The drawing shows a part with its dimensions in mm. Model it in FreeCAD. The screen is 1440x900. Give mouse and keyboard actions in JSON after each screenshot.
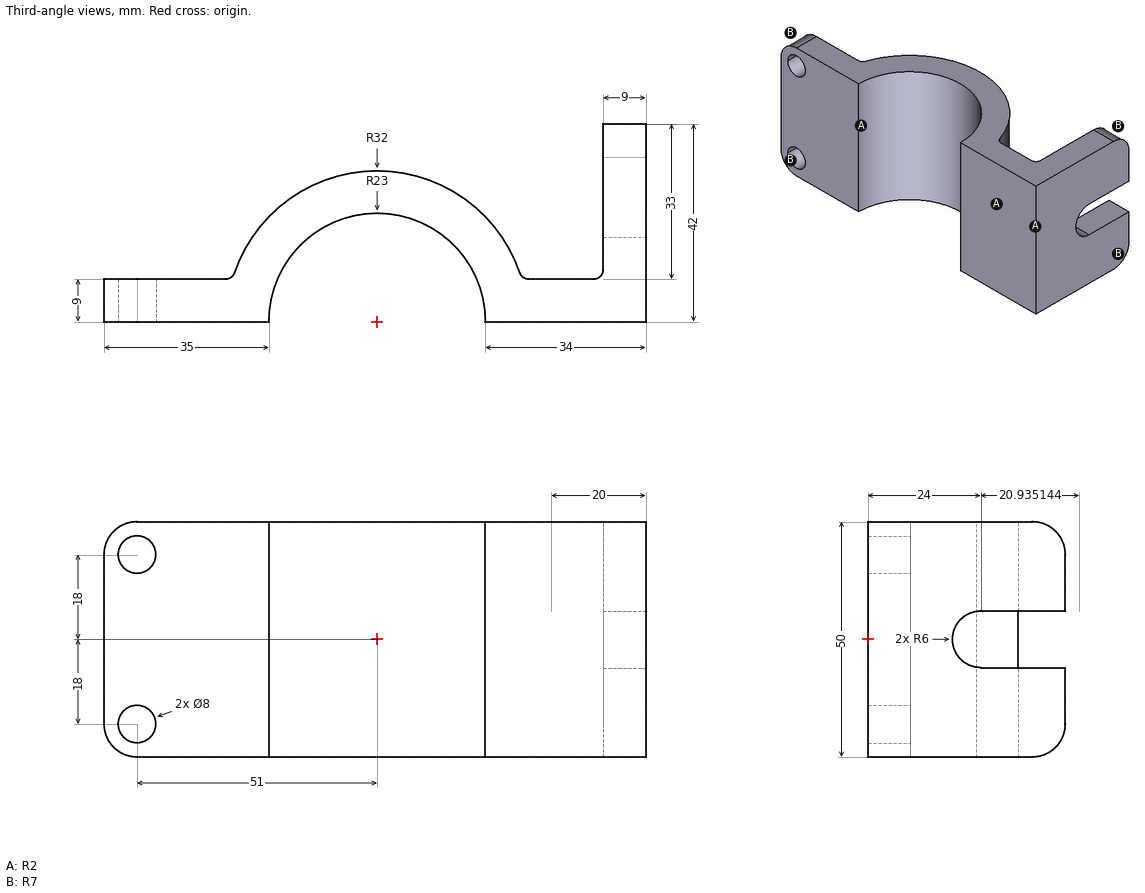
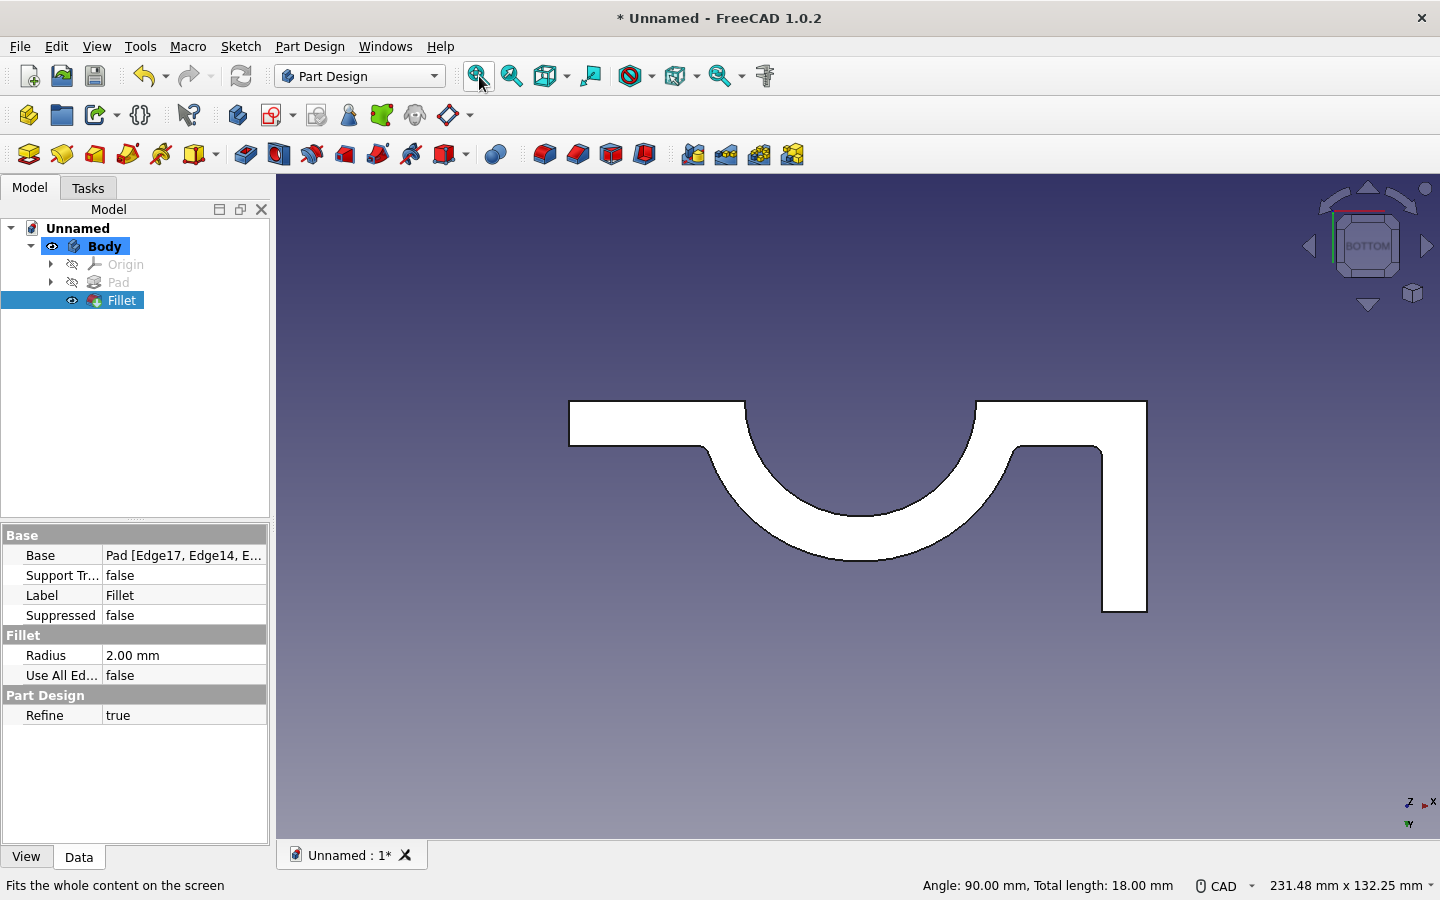
{"action": "left_click", "coordinate": [569, 423], "text": "ctrl"}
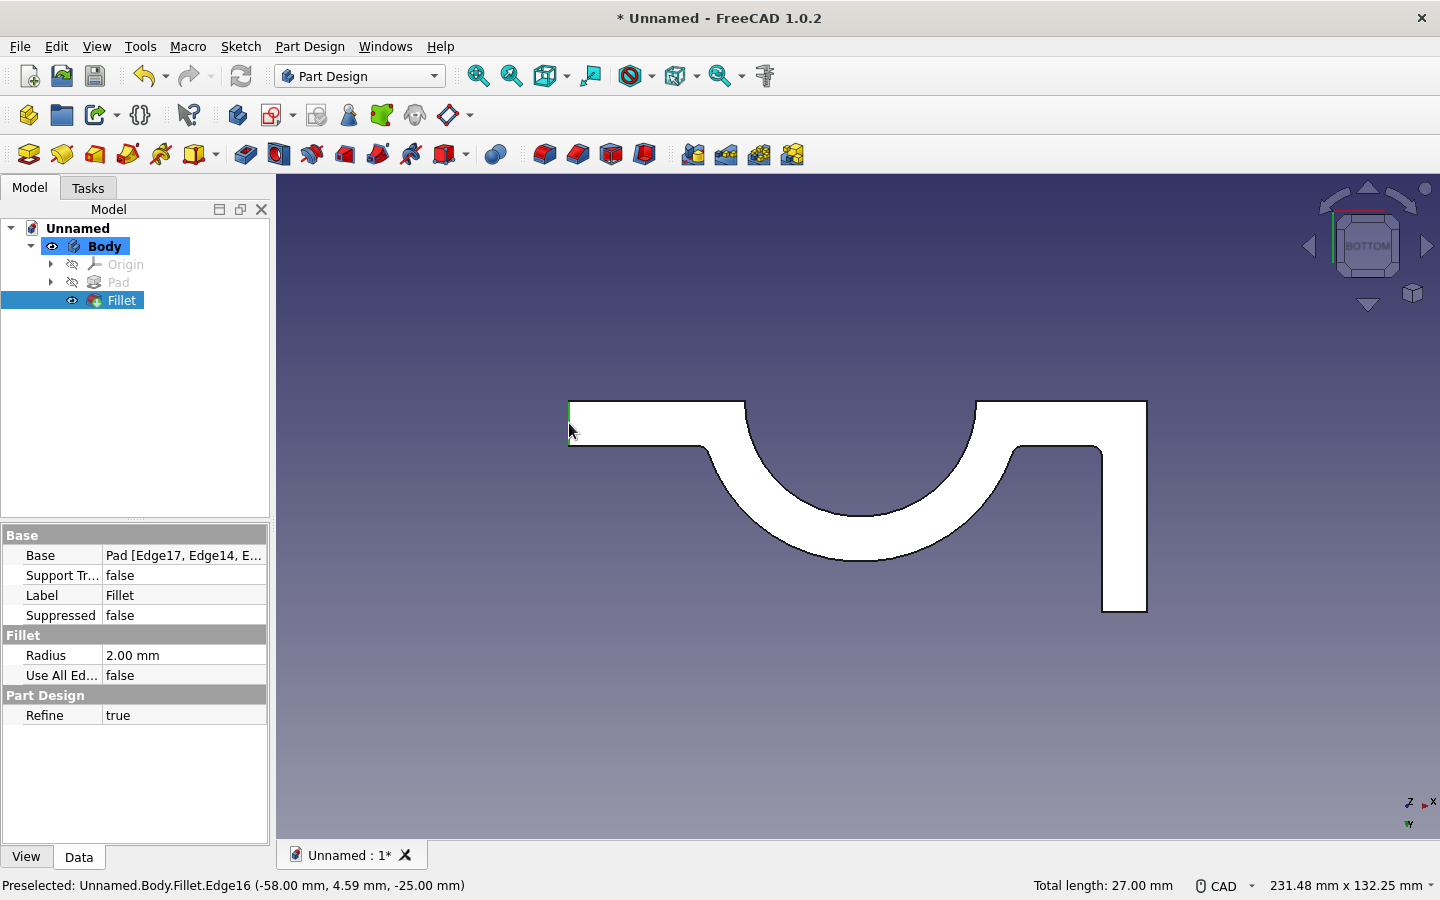
{"action": "left_click", "coordinate": [1125, 611], "text": "ctrl"}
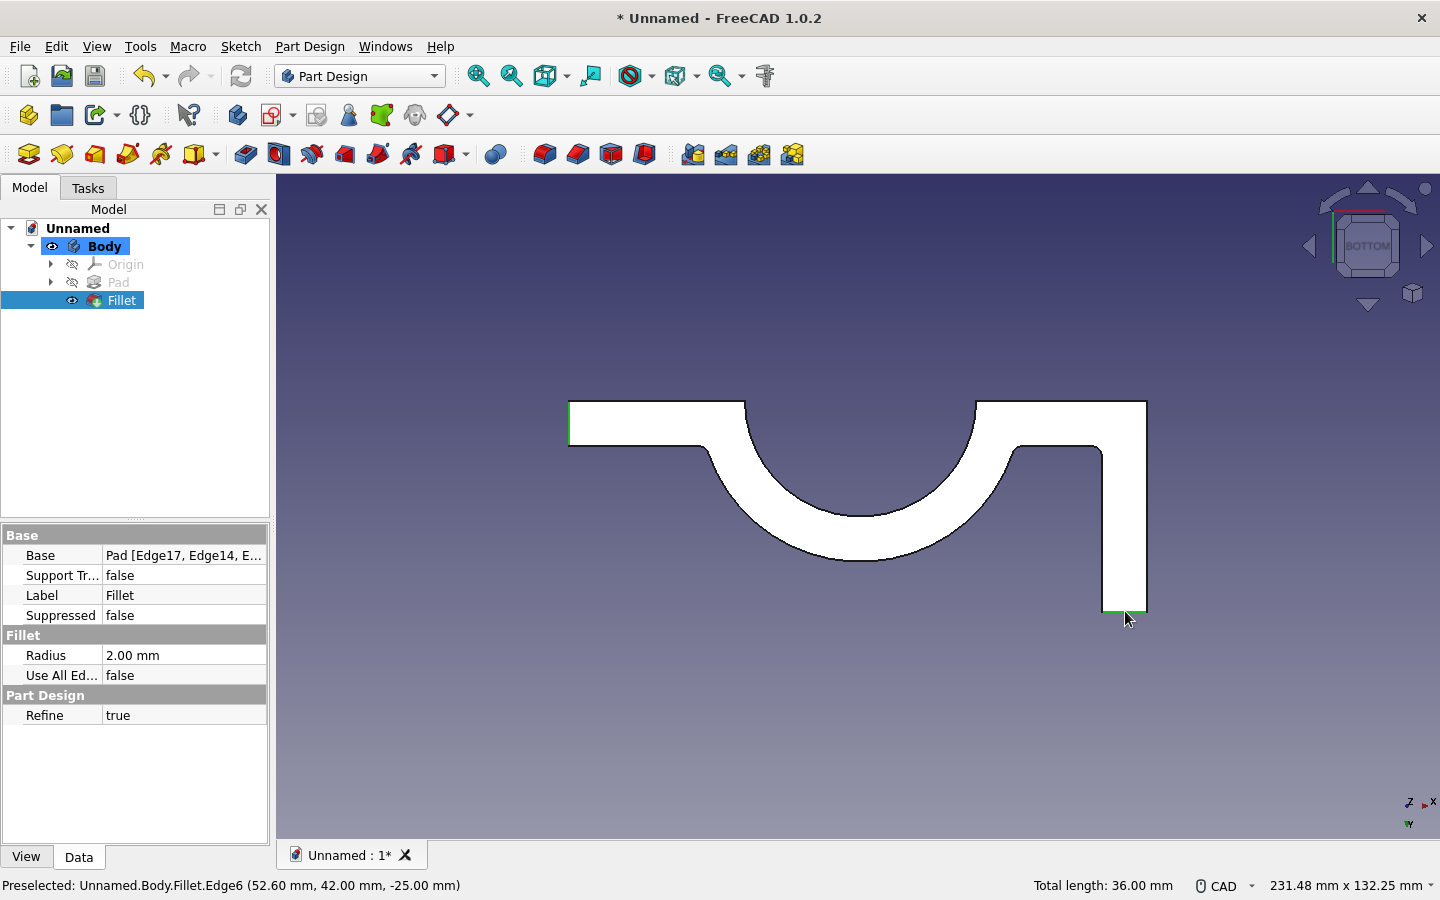
{"action": "left_click", "coordinate": [545, 154]}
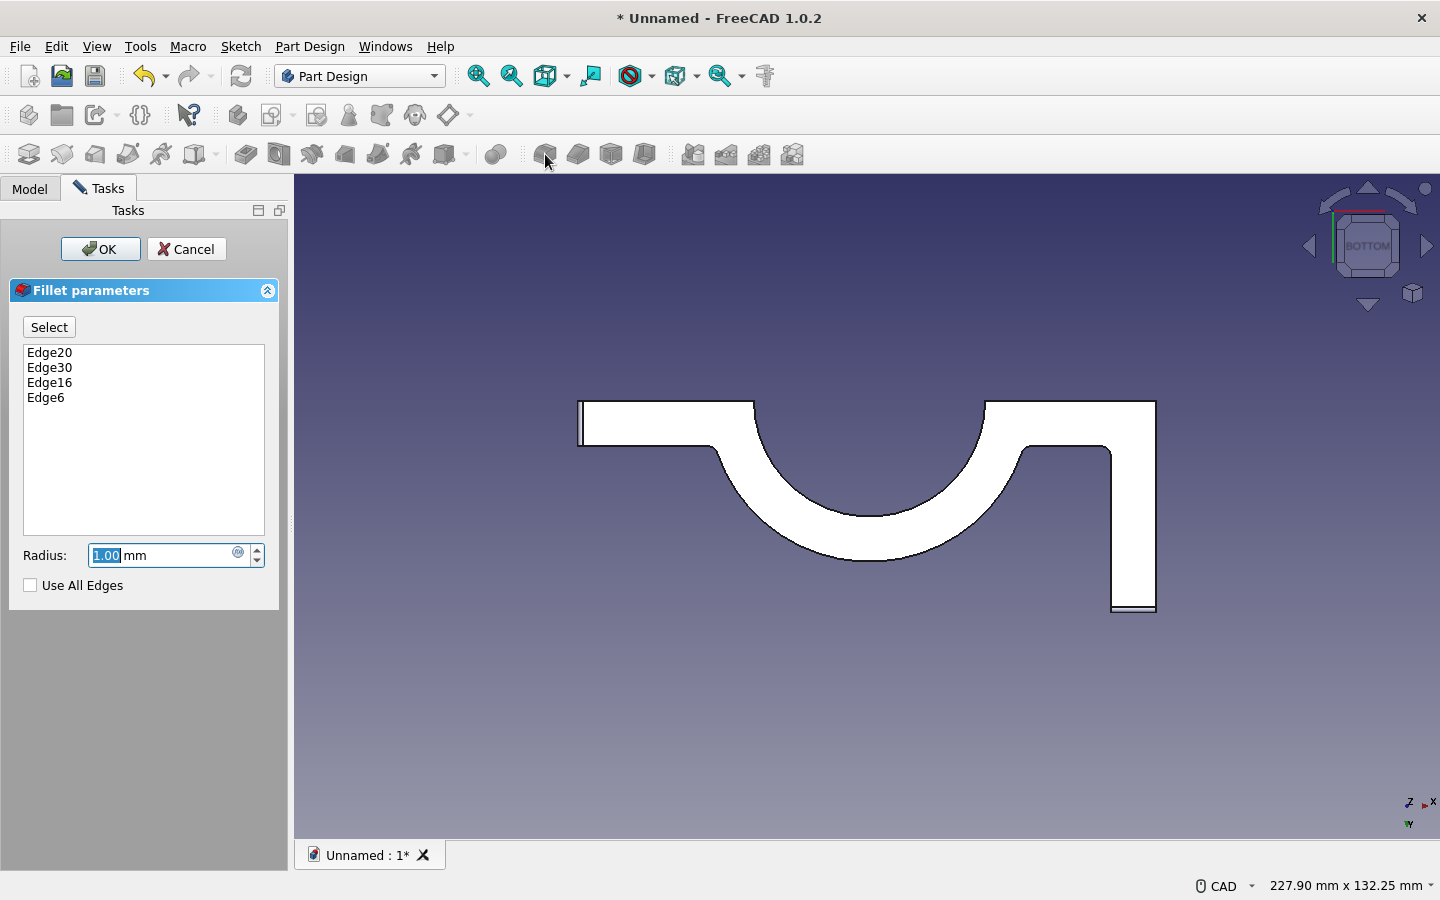
{"action": "type", "text": "7"}
{"action": "key", "text": "Tab"}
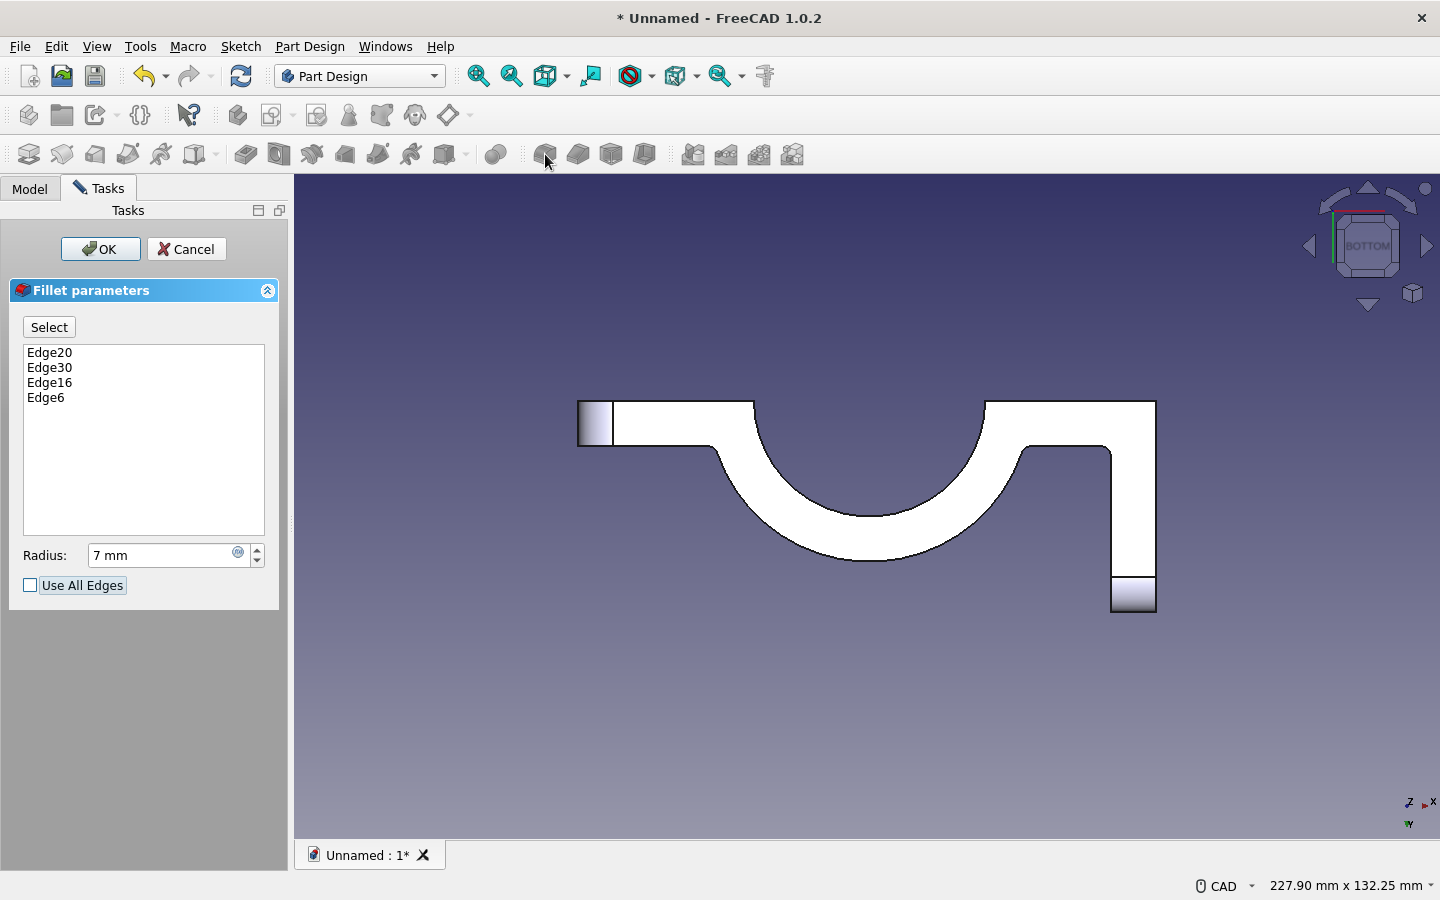
{"action": "left_click", "coordinate": [101, 249]}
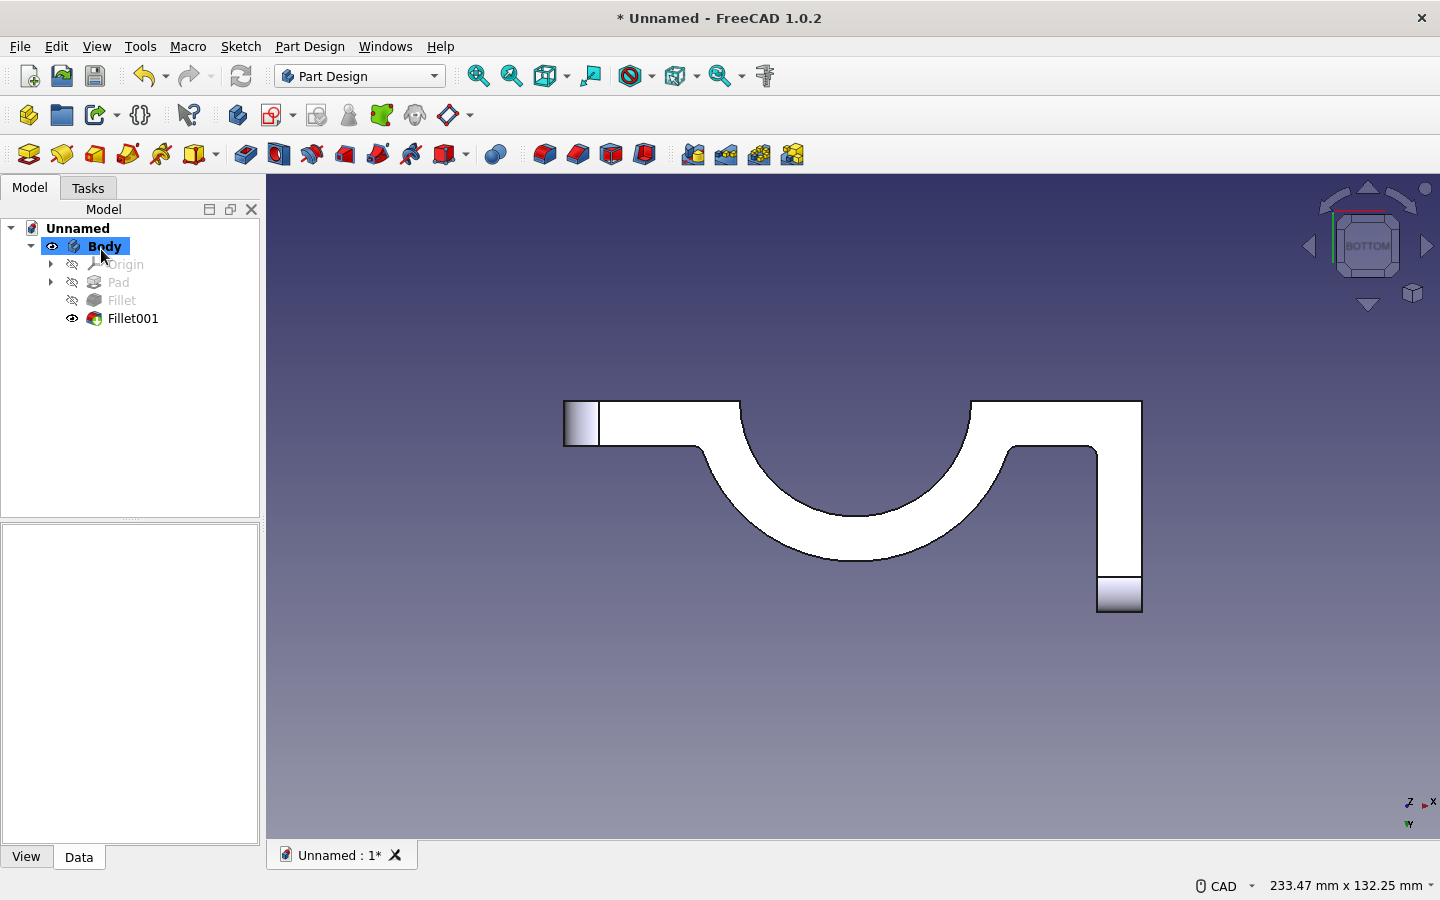
{"action": "key", "text": "4"}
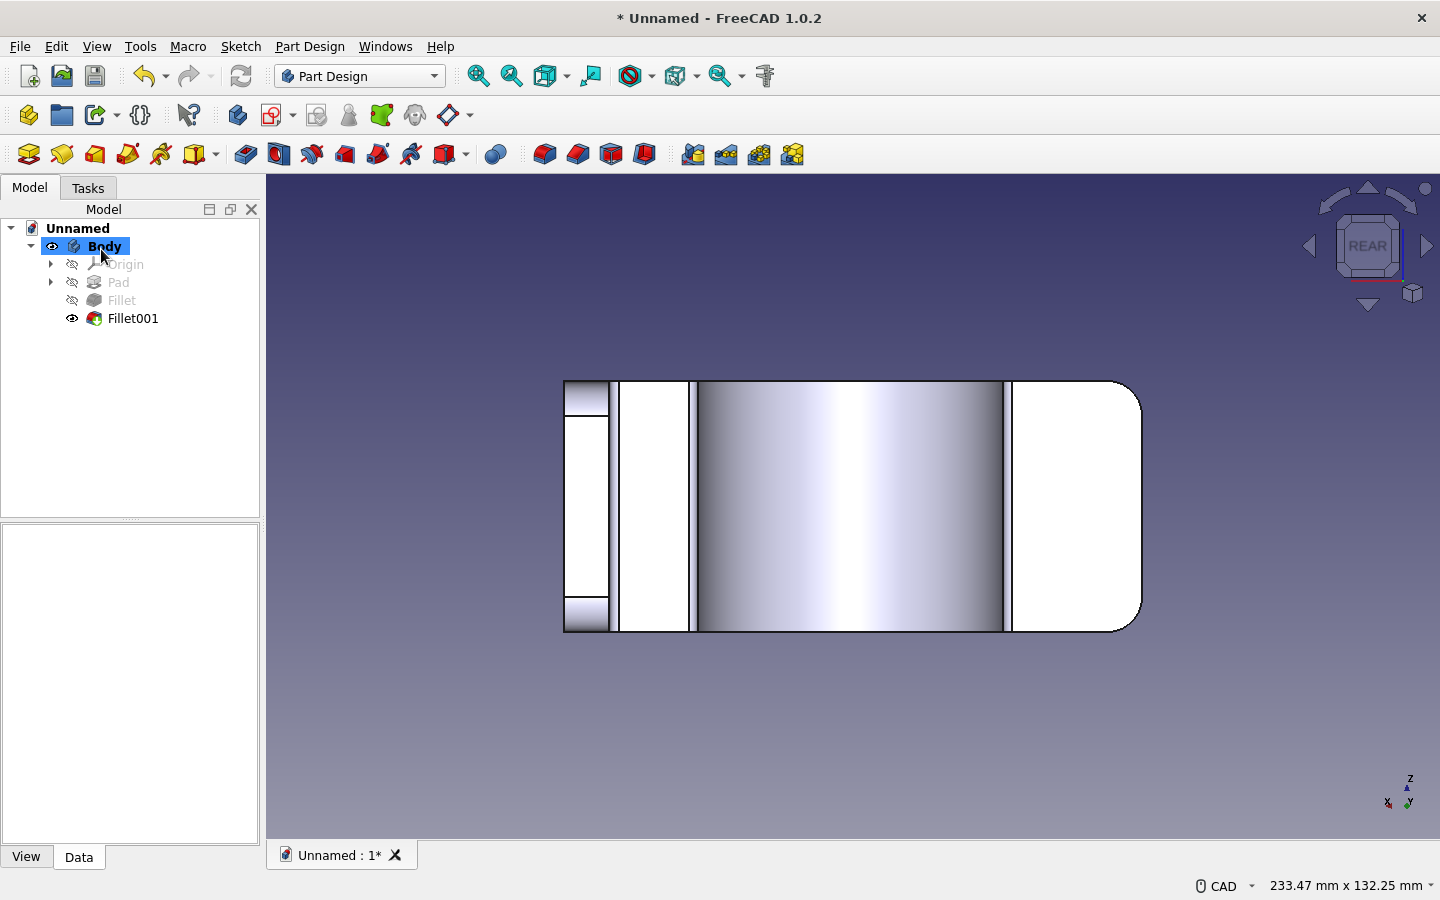
{"action": "left_click", "coordinate": [1077, 470]}